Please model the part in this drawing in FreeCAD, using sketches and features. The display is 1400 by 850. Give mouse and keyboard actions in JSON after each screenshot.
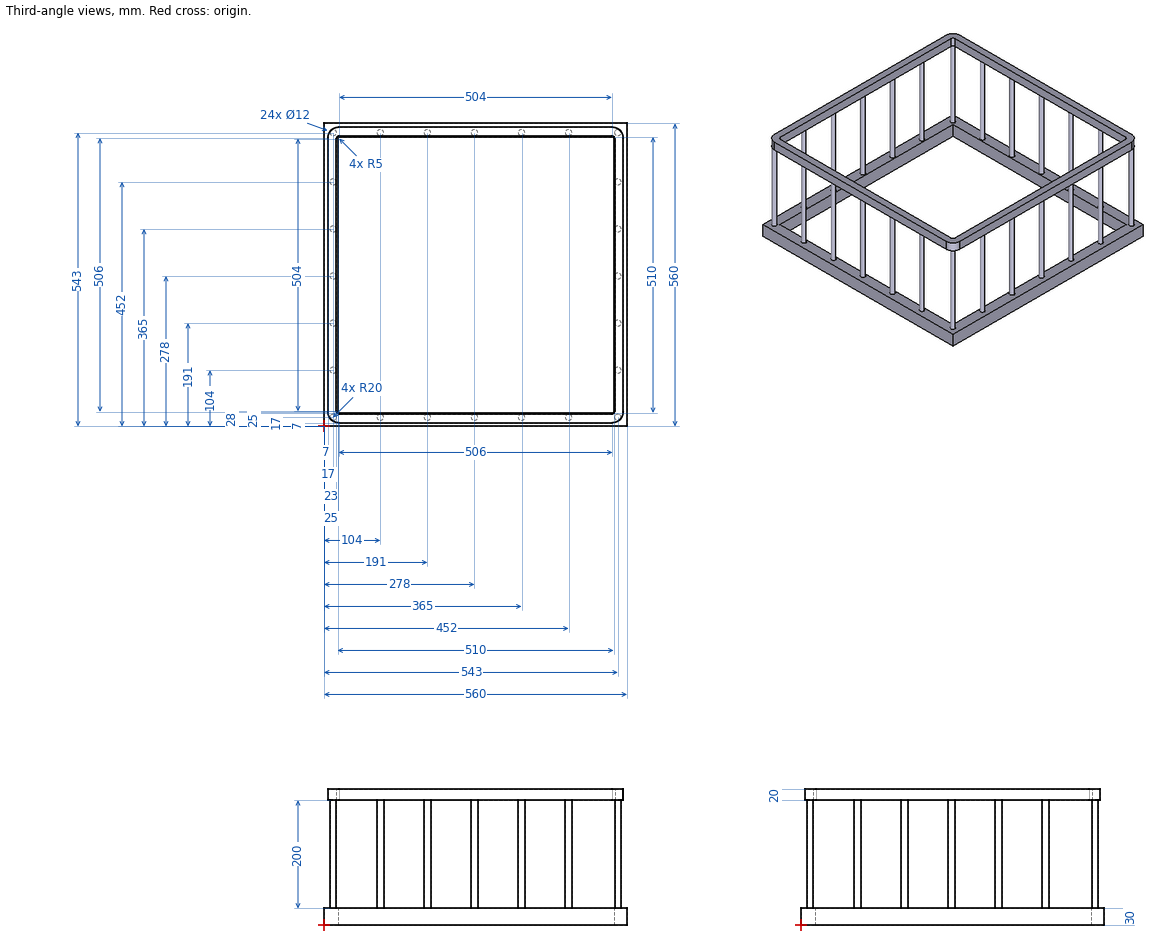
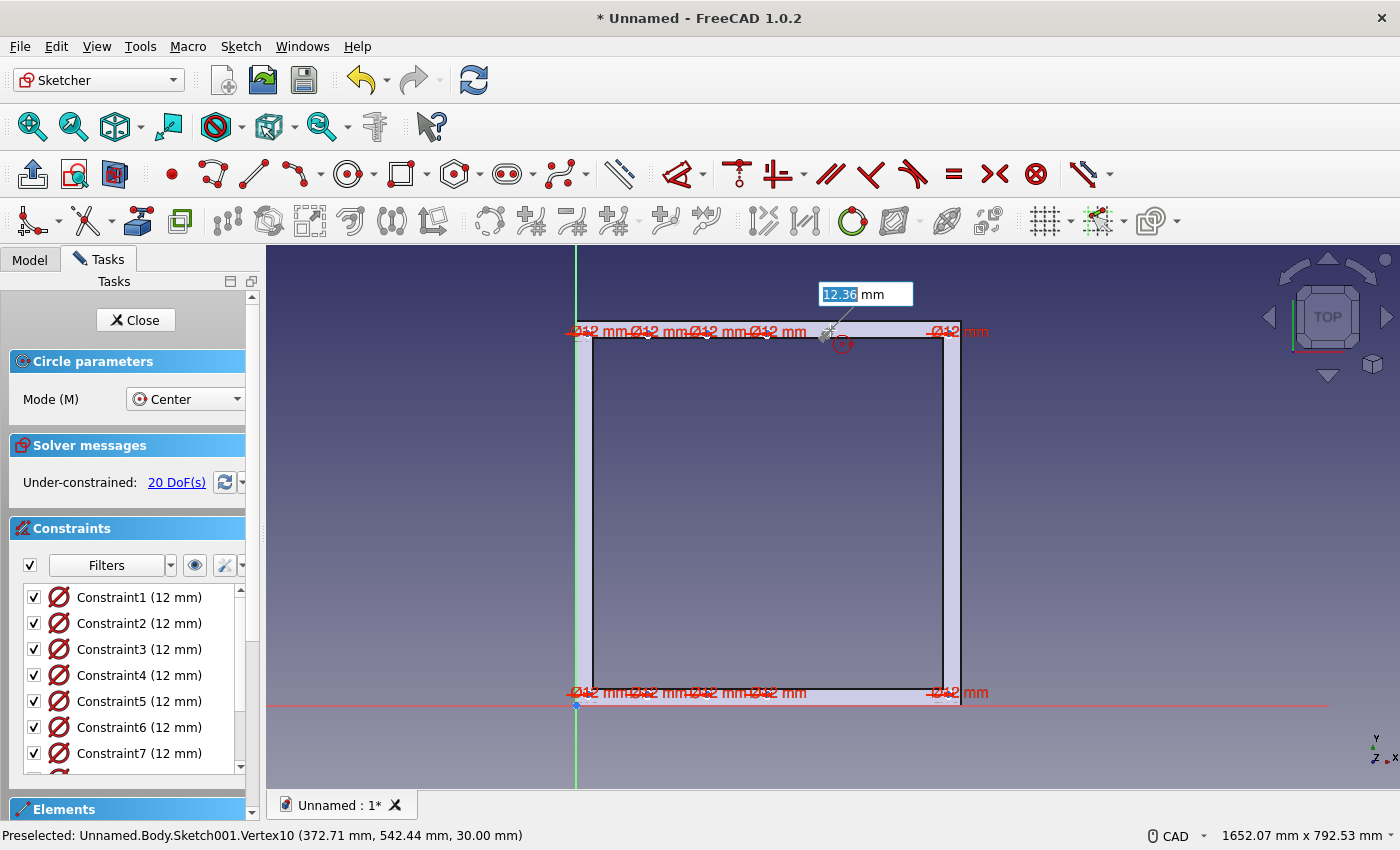
{"action": "type", "text": "12"}
{"action": "key", "text": "Return"}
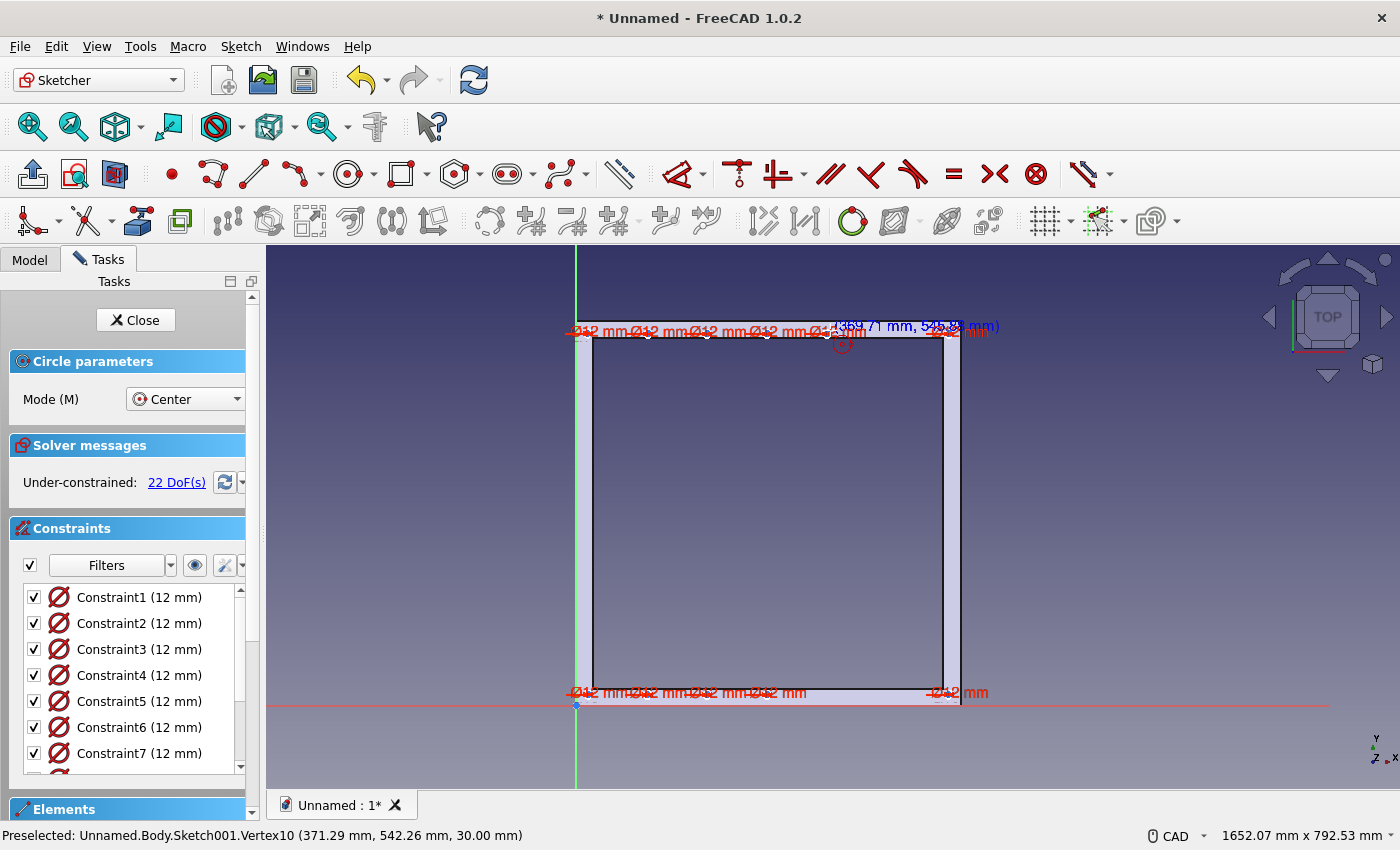
{"action": "scroll", "coordinate": [827, 694], "scroll_direction": "up", "scroll_amount": 9}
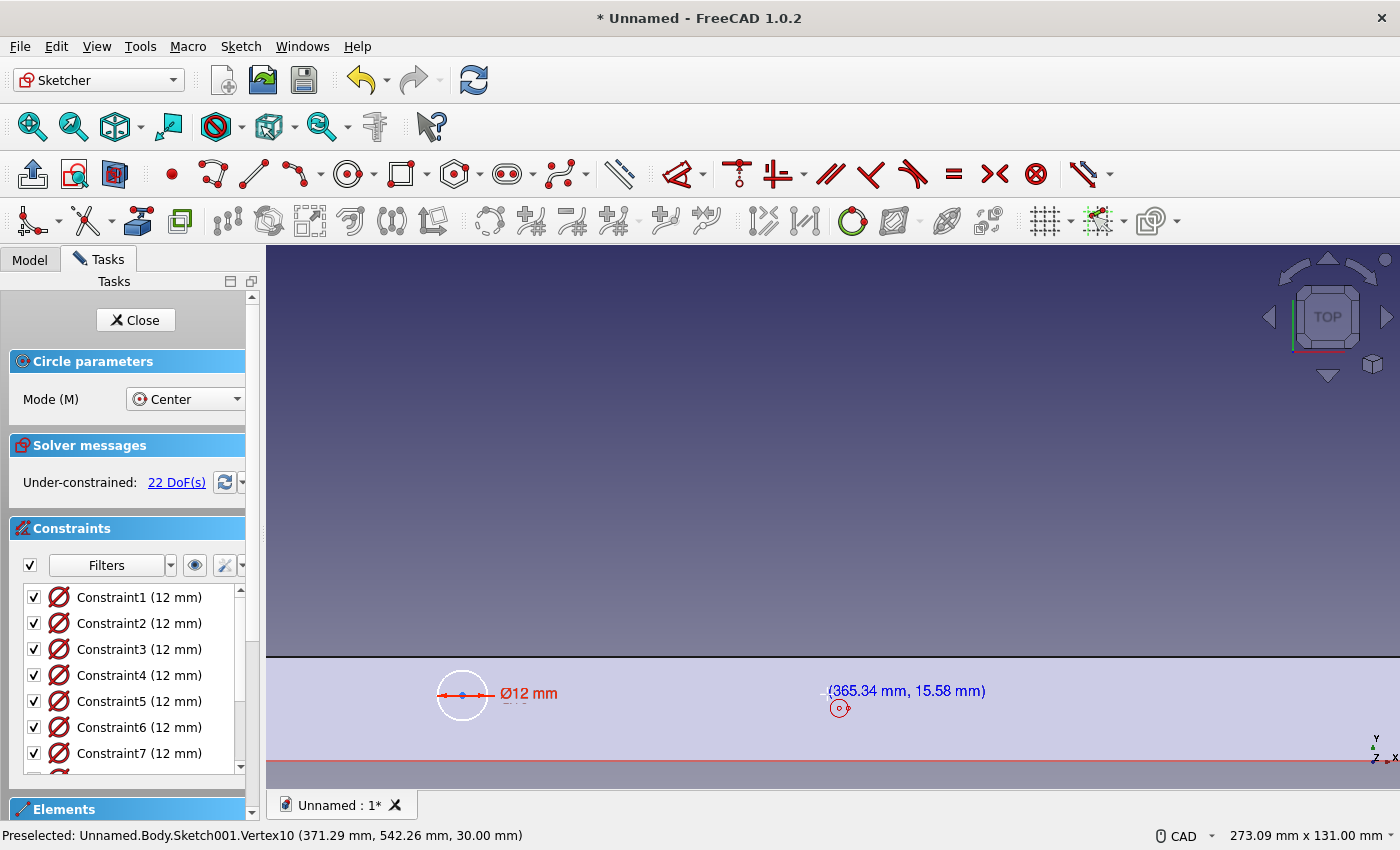
{"action": "scroll", "coordinate": [827, 694], "scroll_direction": "down", "scroll_amount": 9}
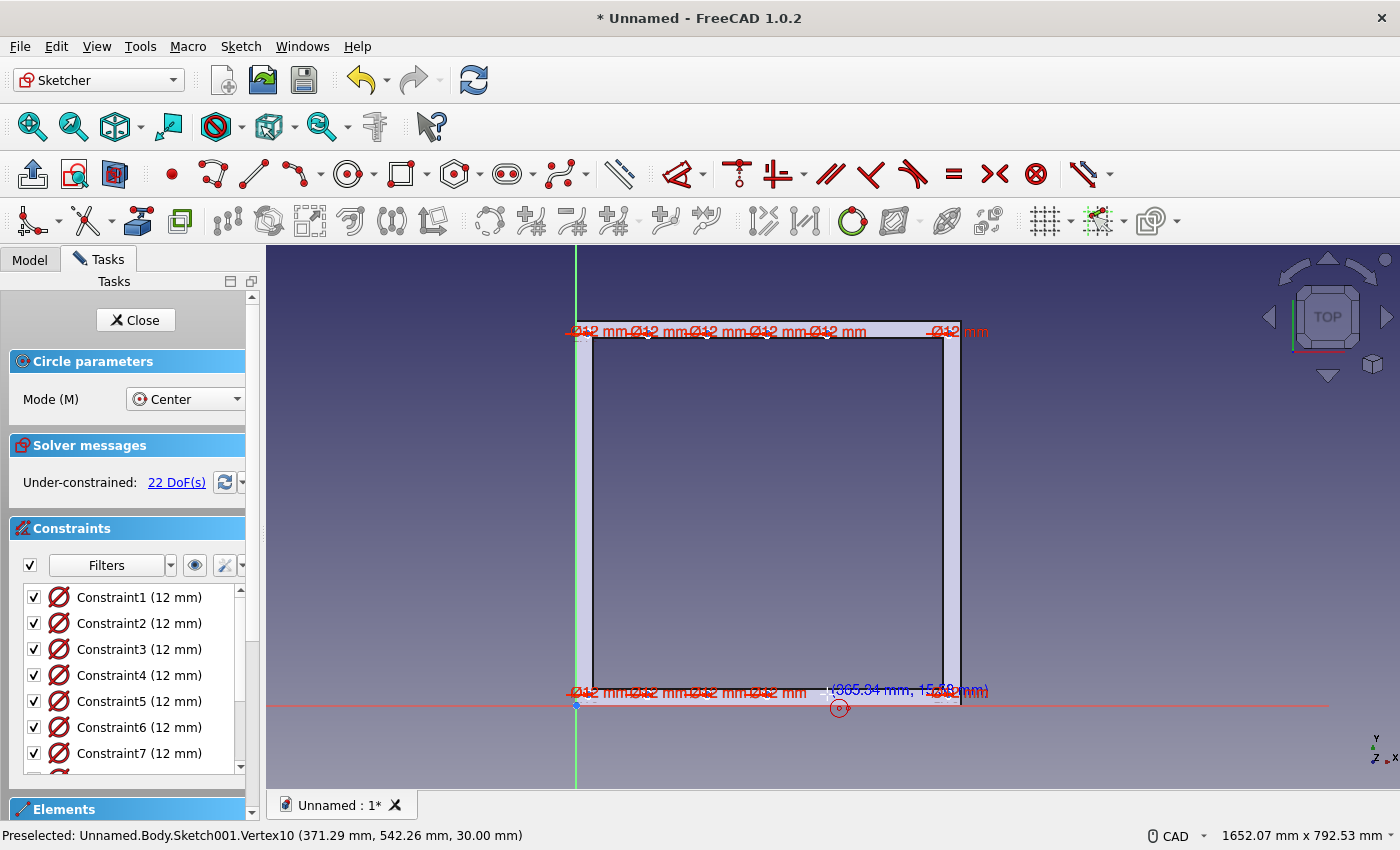
{"action": "scroll", "coordinate": [827, 694], "scroll_direction": "up", "scroll_amount": 2}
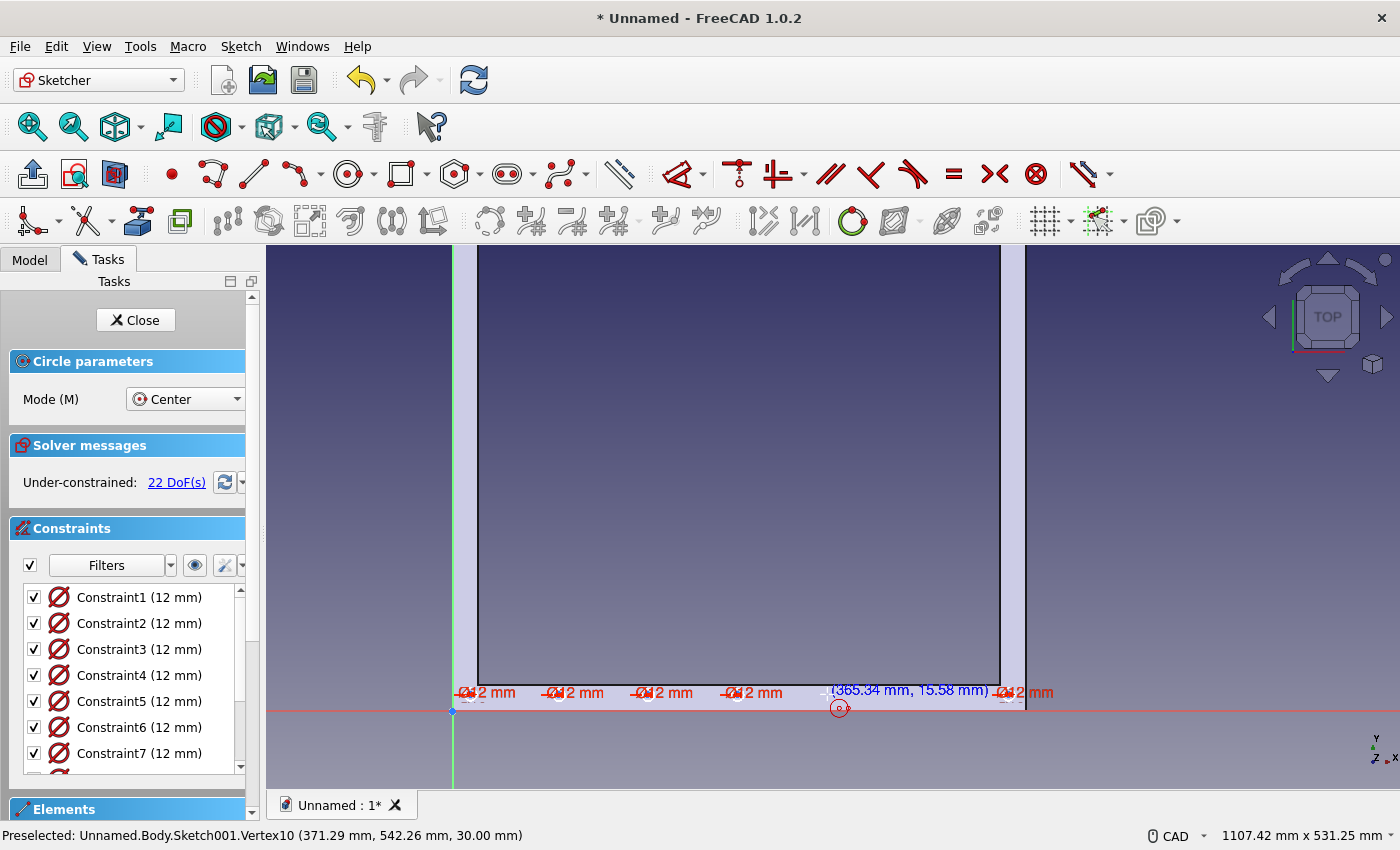
{"action": "left_click", "coordinate": [826, 694]}
{"action": "mouse_move", "coordinate": [831, 689]}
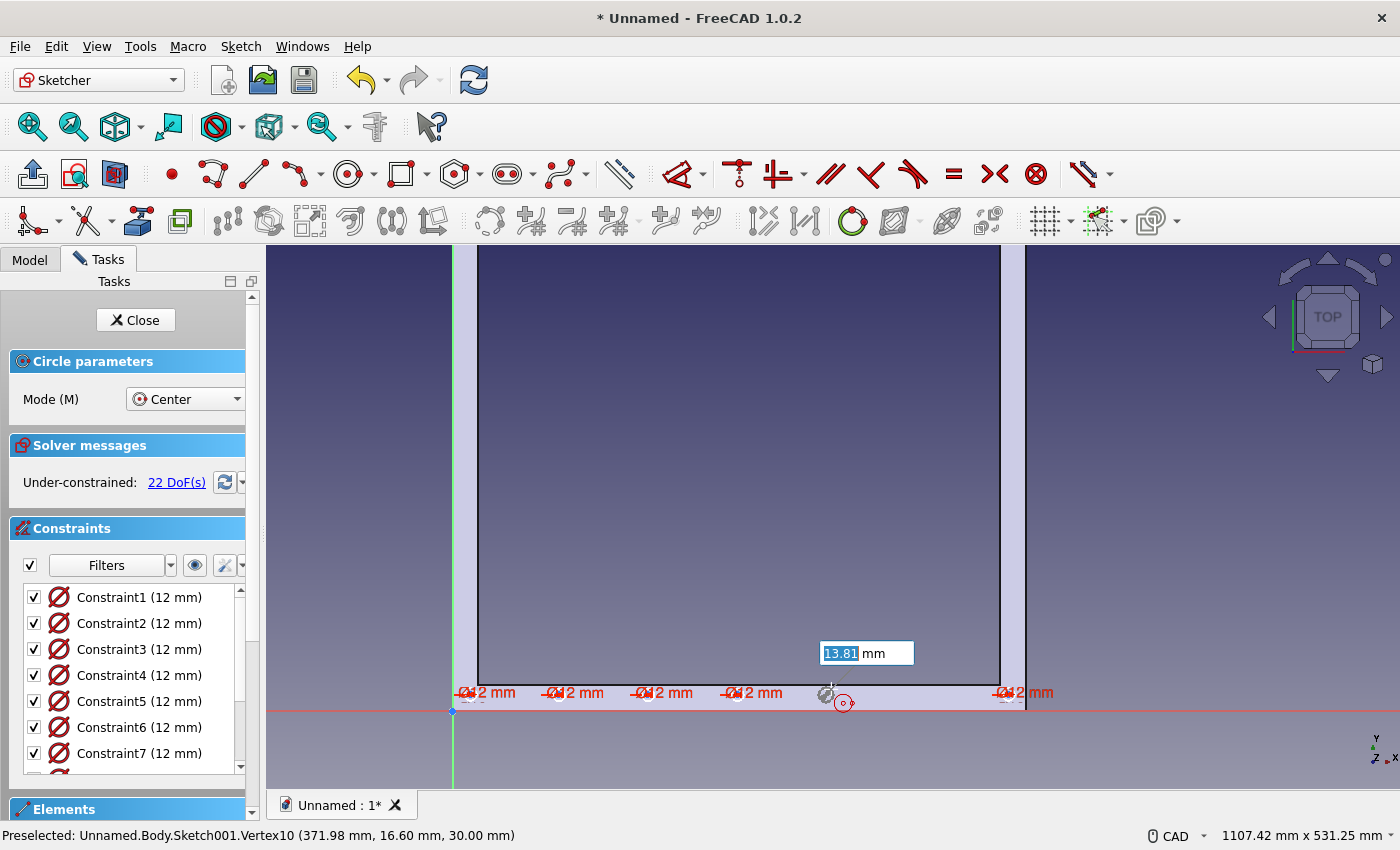
{"action": "type", "text": "12"}
{"action": "key", "text": "Return"}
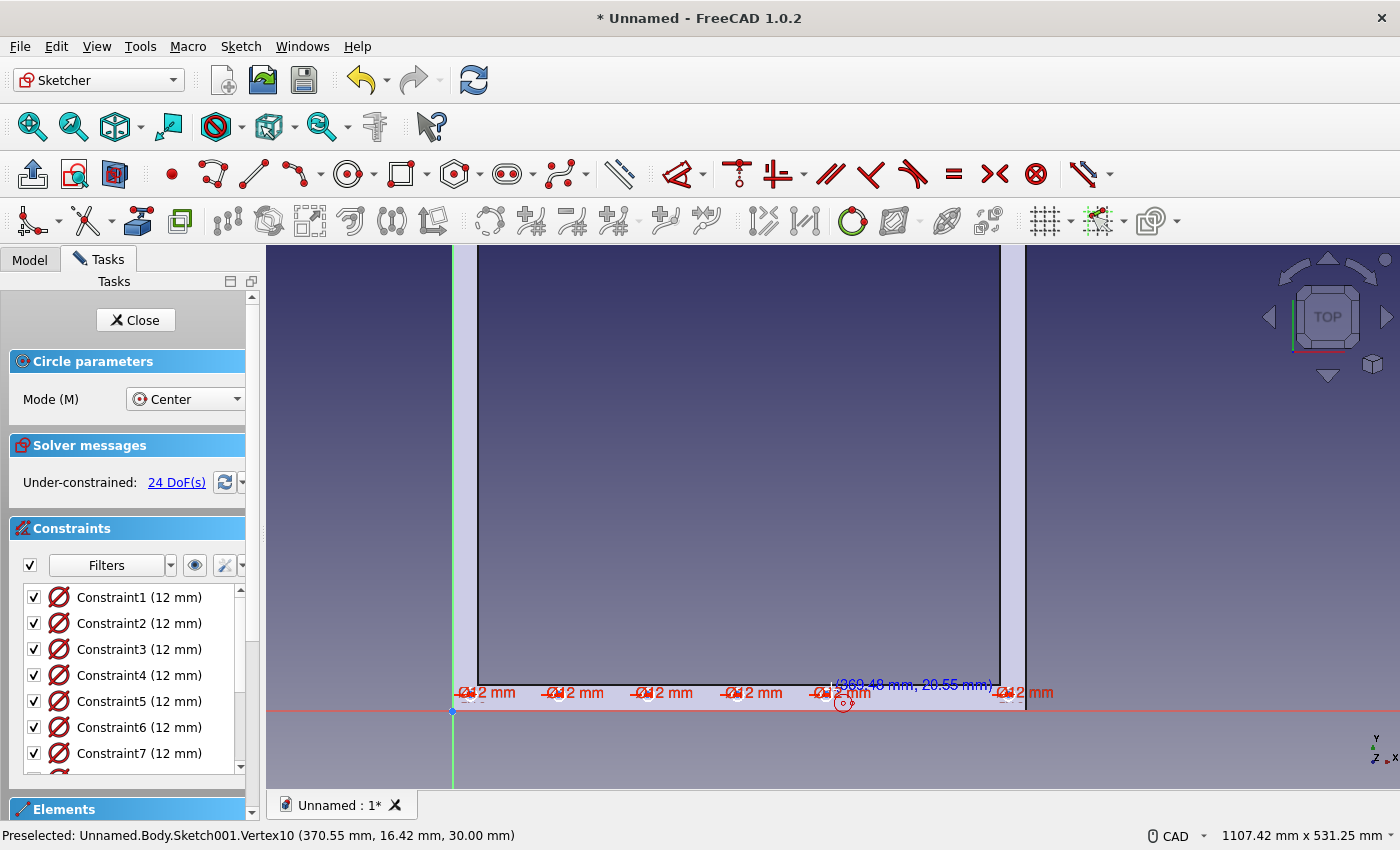
{"action": "scroll", "coordinate": [827, 694], "scroll_direction": "down", "scroll_amount": 2}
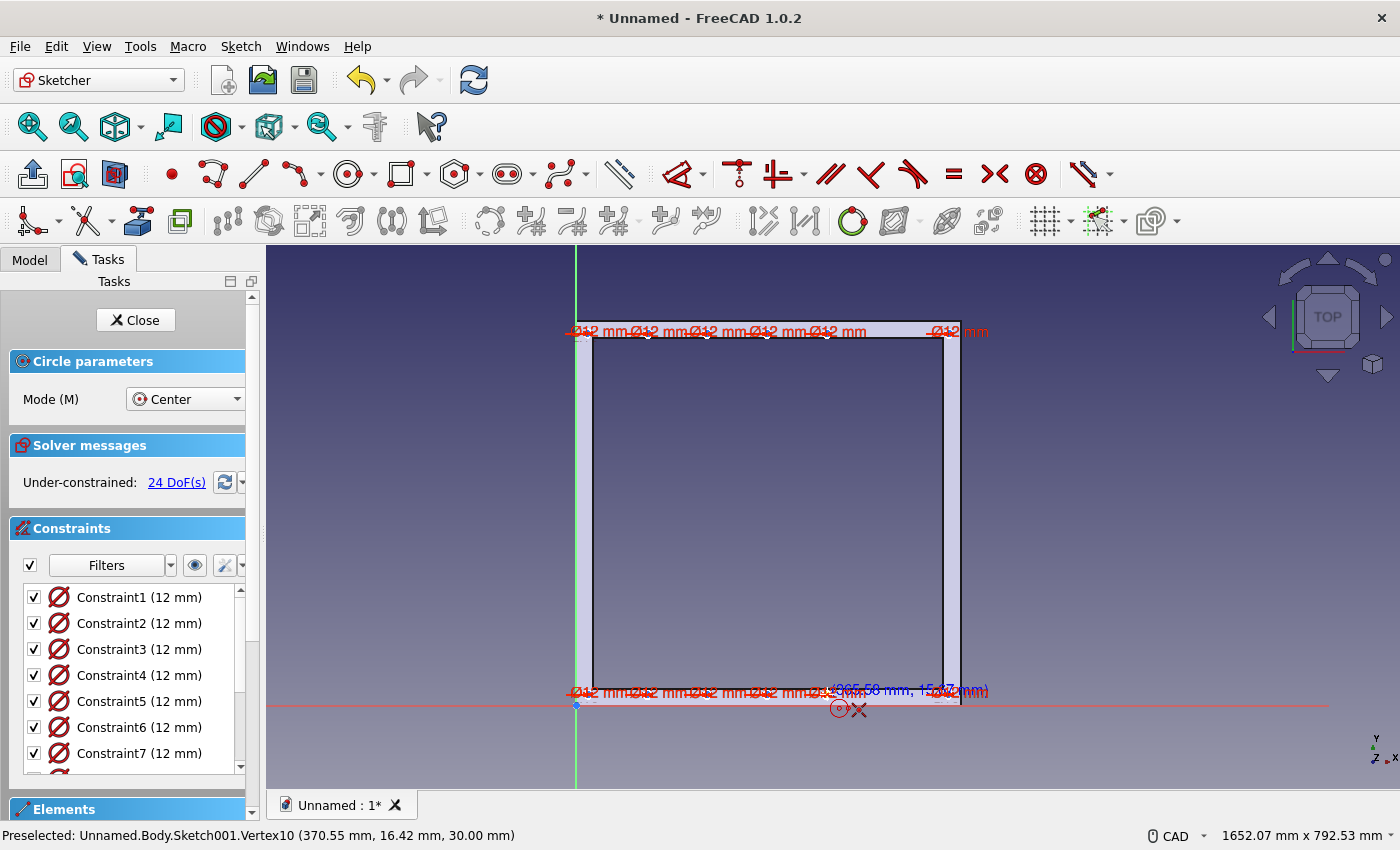
{"action": "scroll", "coordinate": [886, 333], "scroll_direction": "up", "scroll_amount": 9}